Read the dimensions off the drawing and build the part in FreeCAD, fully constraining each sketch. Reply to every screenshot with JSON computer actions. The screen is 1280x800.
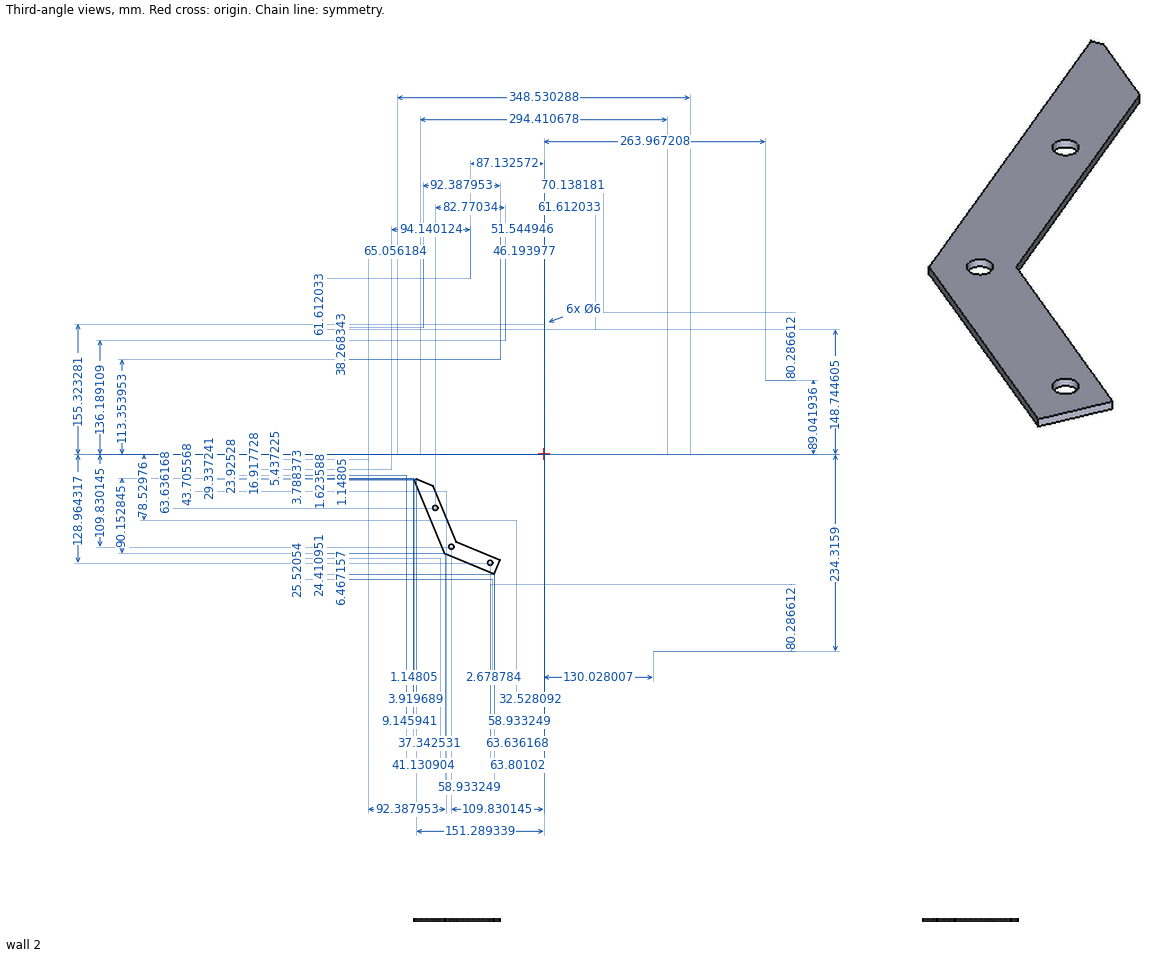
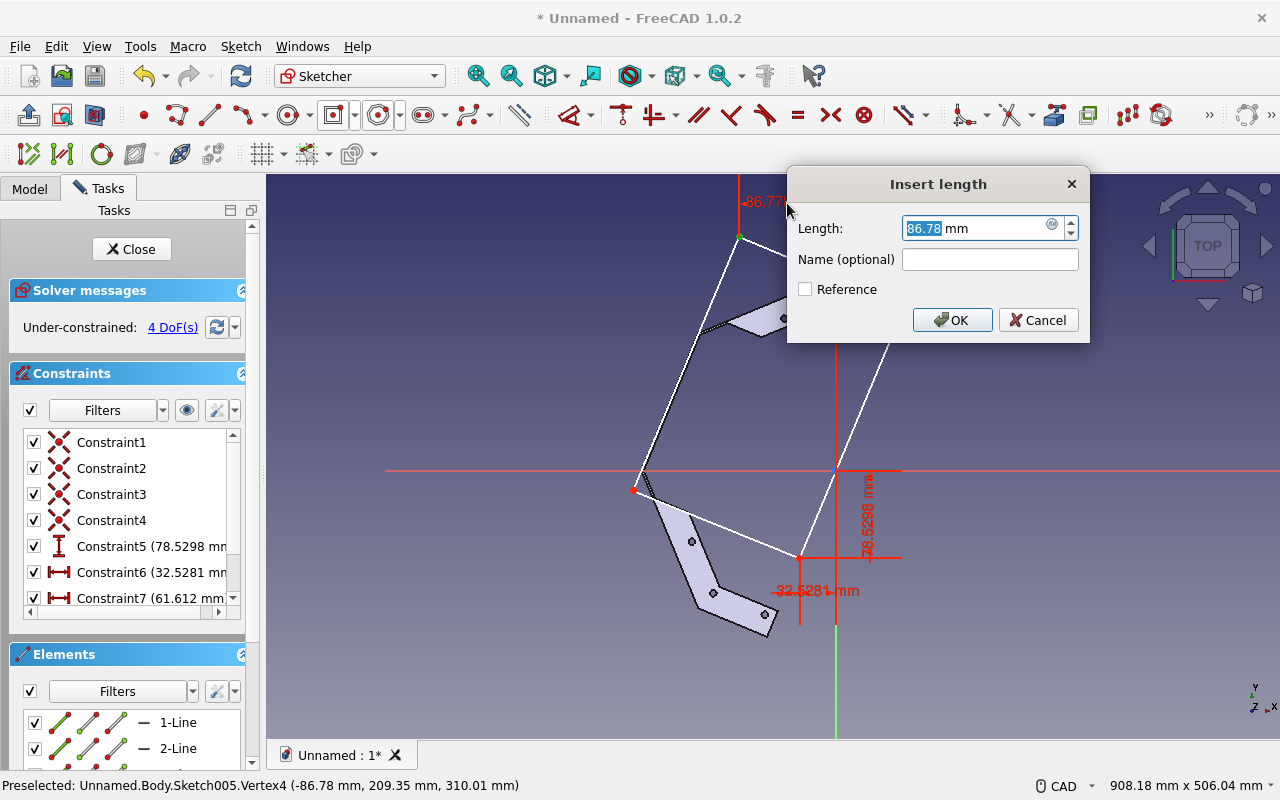
{"action": "type", "text": "87.132572"}
{"action": "key", "text": "Return"}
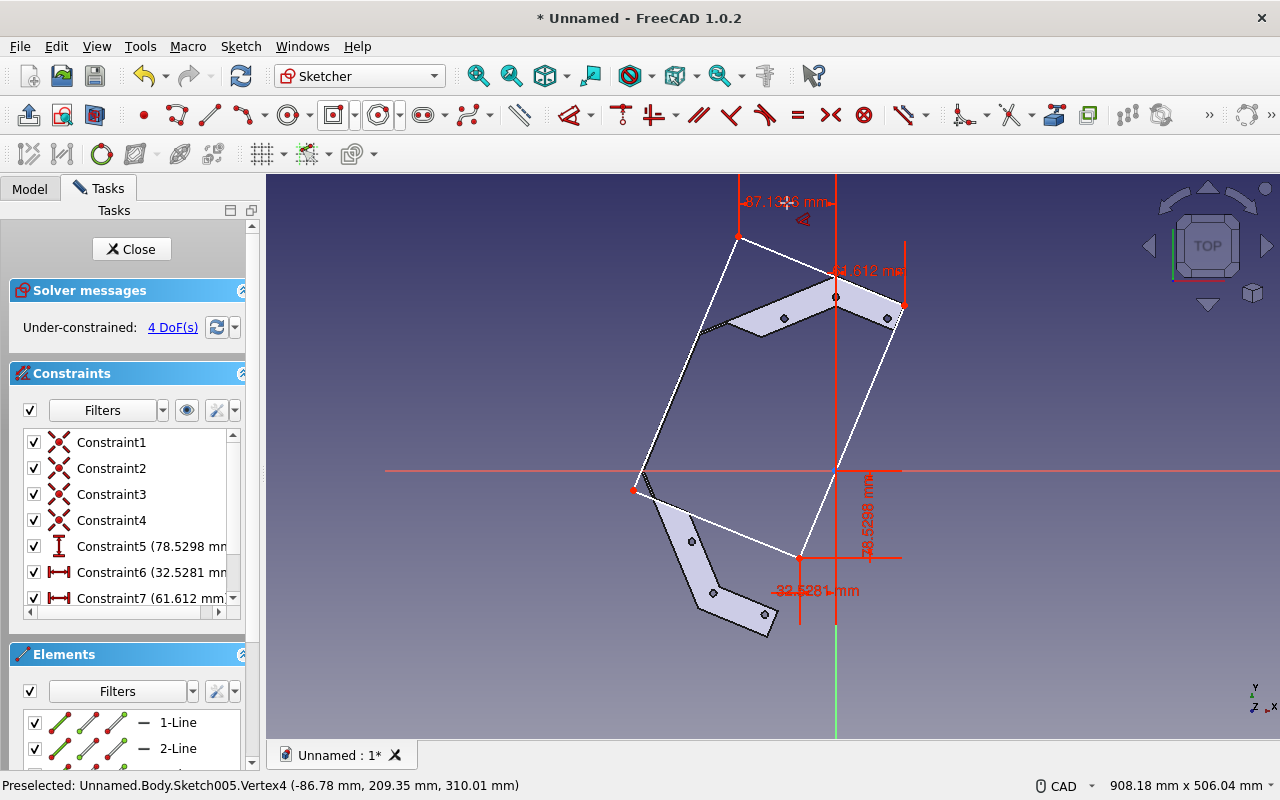
{"action": "scroll", "coordinate": [633, 491], "scroll_direction": "up", "scroll_amount": 4}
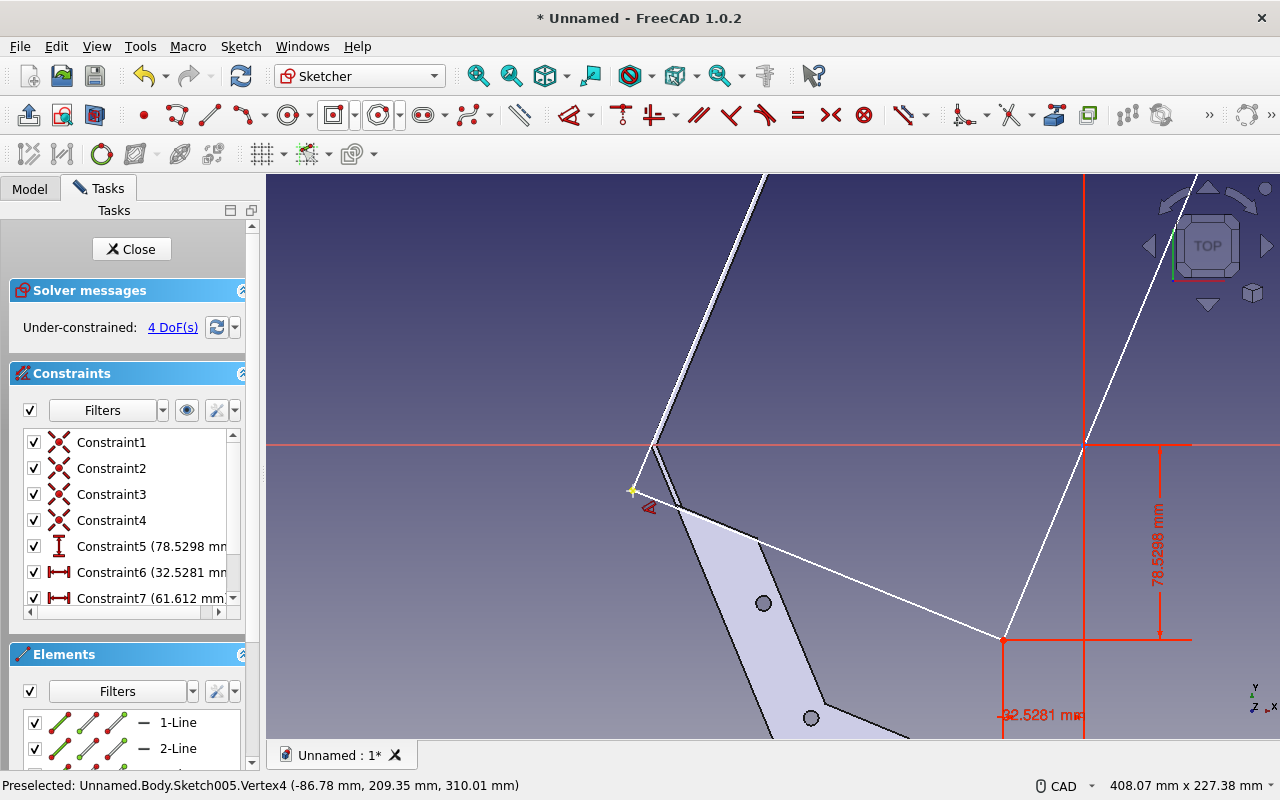
{"action": "left_click", "coordinate": [633, 490]}
{"action": "left_click", "coordinate": [599, 468]}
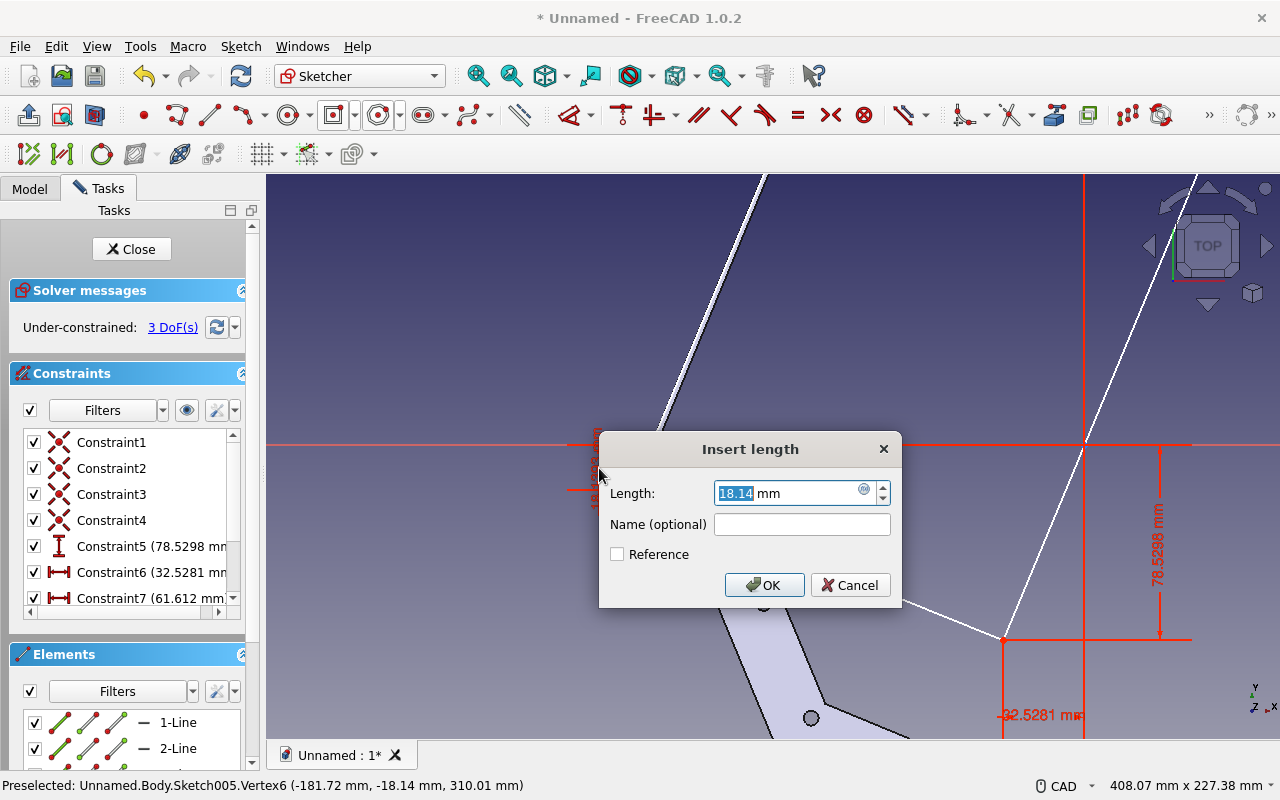
{"action": "type", "text": "16.917728"}
{"action": "key", "text": "Return"}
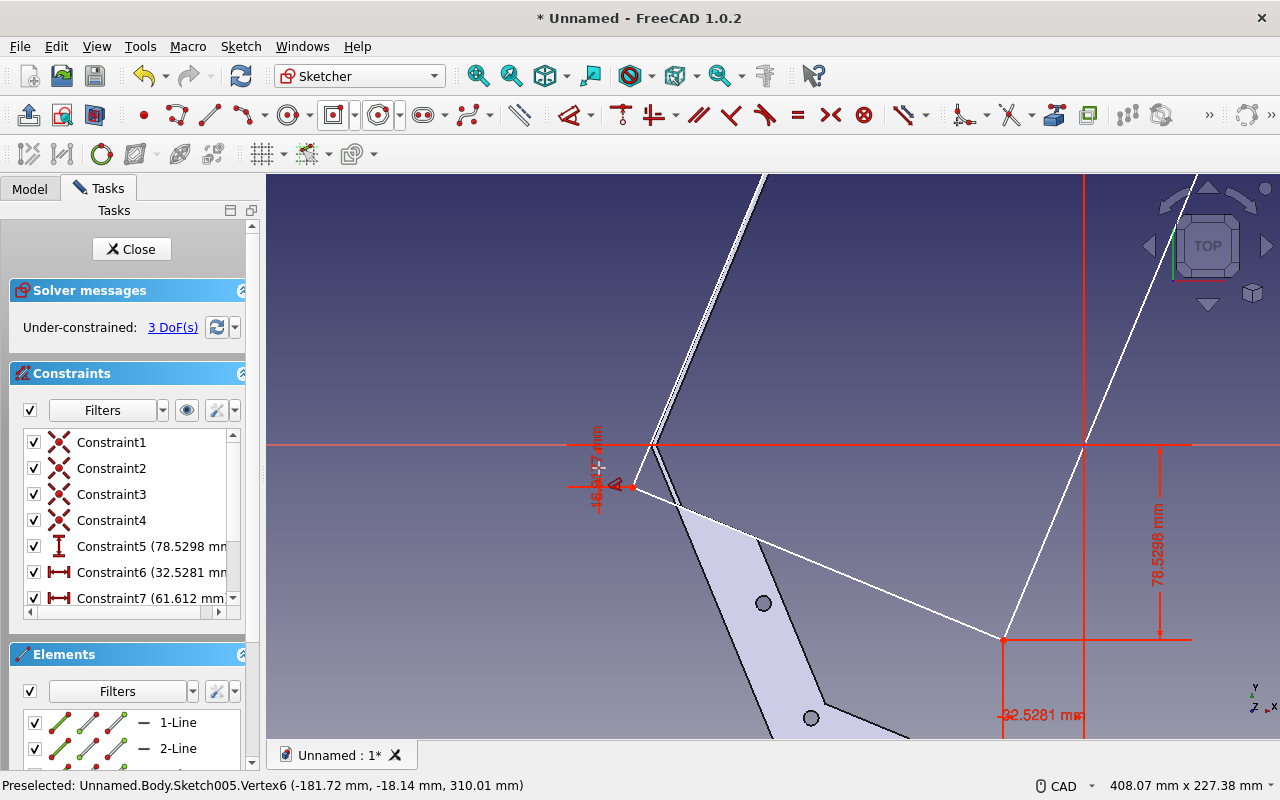
{"action": "scroll", "coordinate": [424, 669], "scroll_direction": "down", "scroll_amount": 3}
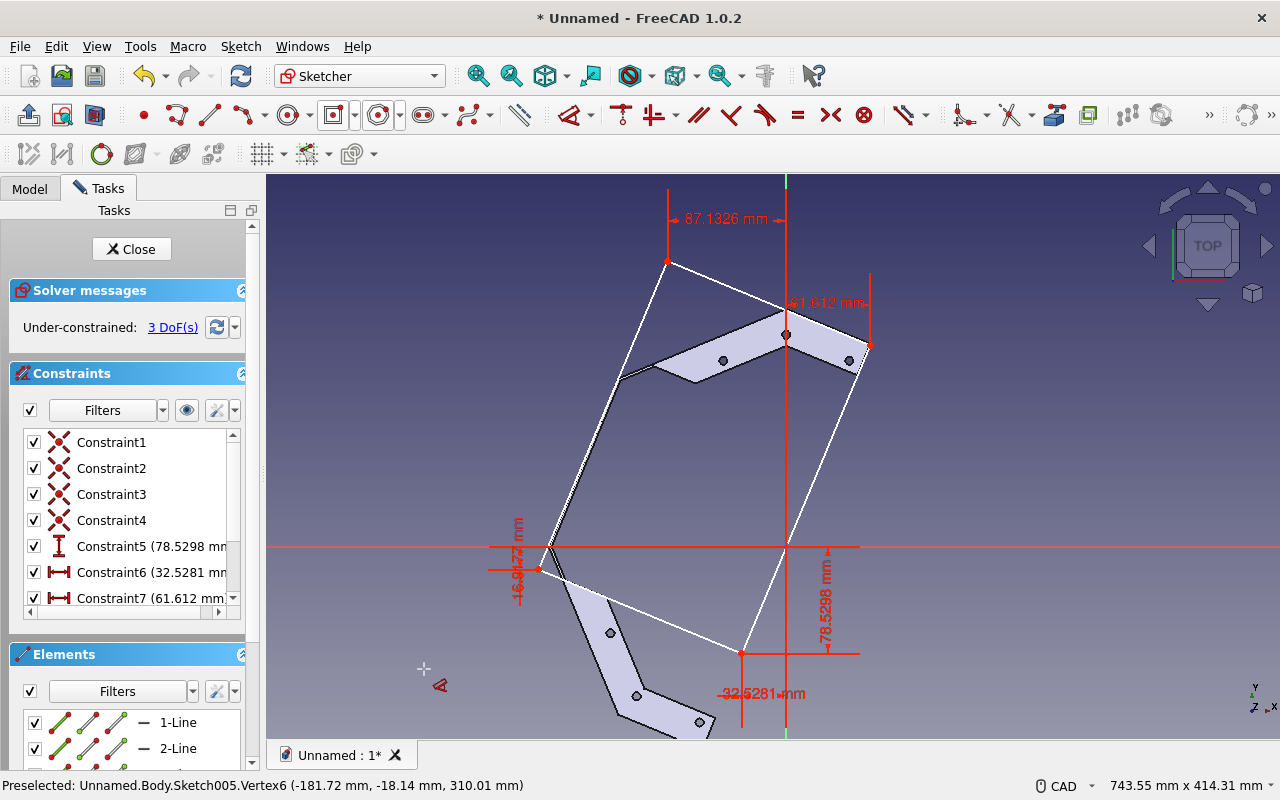
{"action": "left_click", "coordinate": [810, 320]}
{"action": "left_click", "coordinate": [904, 303]}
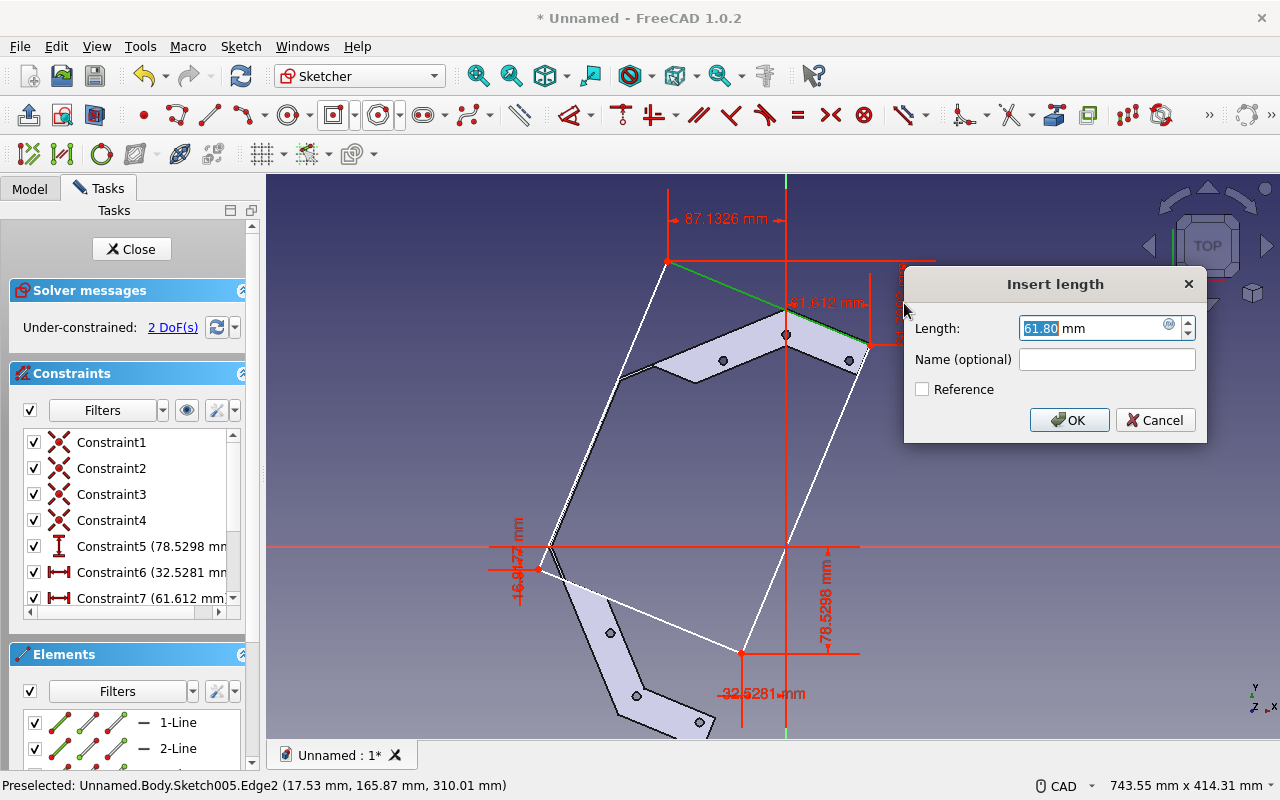
{"action": "type", "text": "61.612033"}
{"action": "key", "text": "Return"}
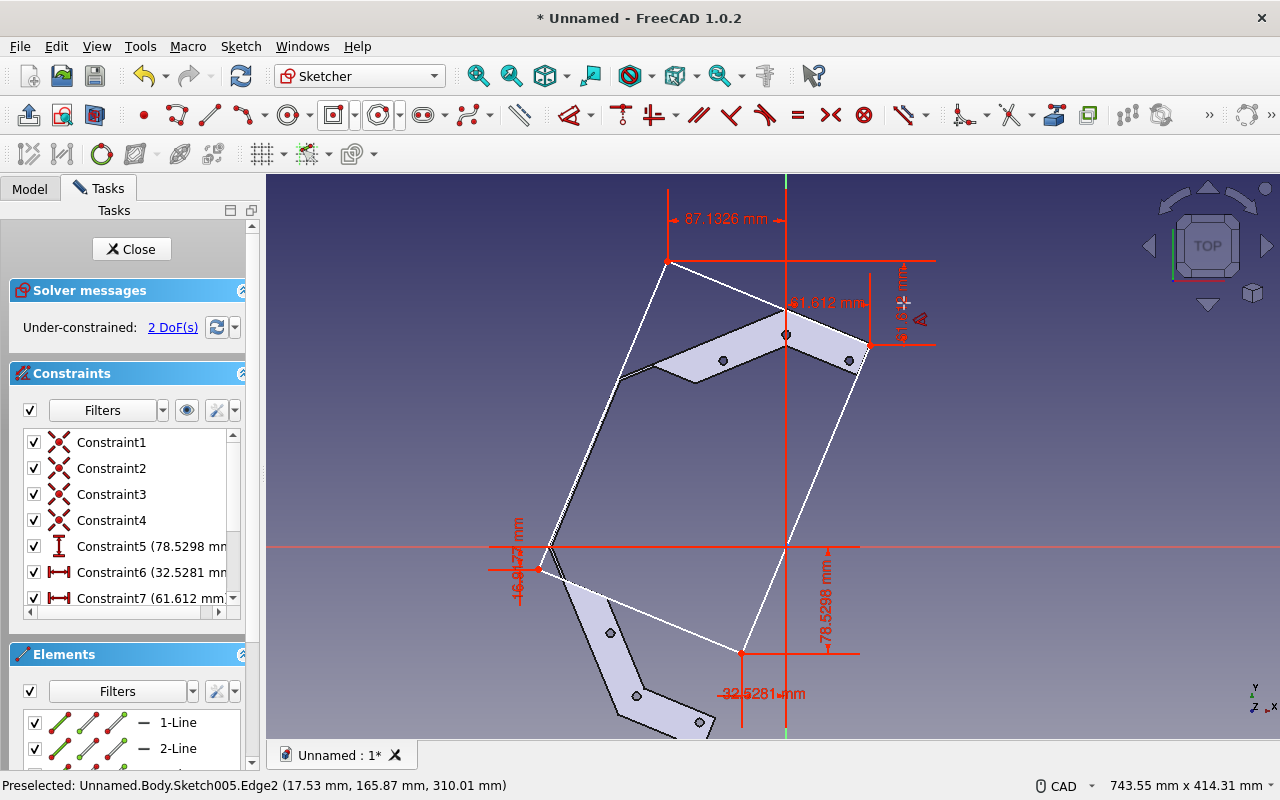
{"action": "left_click", "coordinate": [629, 354]}
{"action": "left_click", "coordinate": [603, 227]}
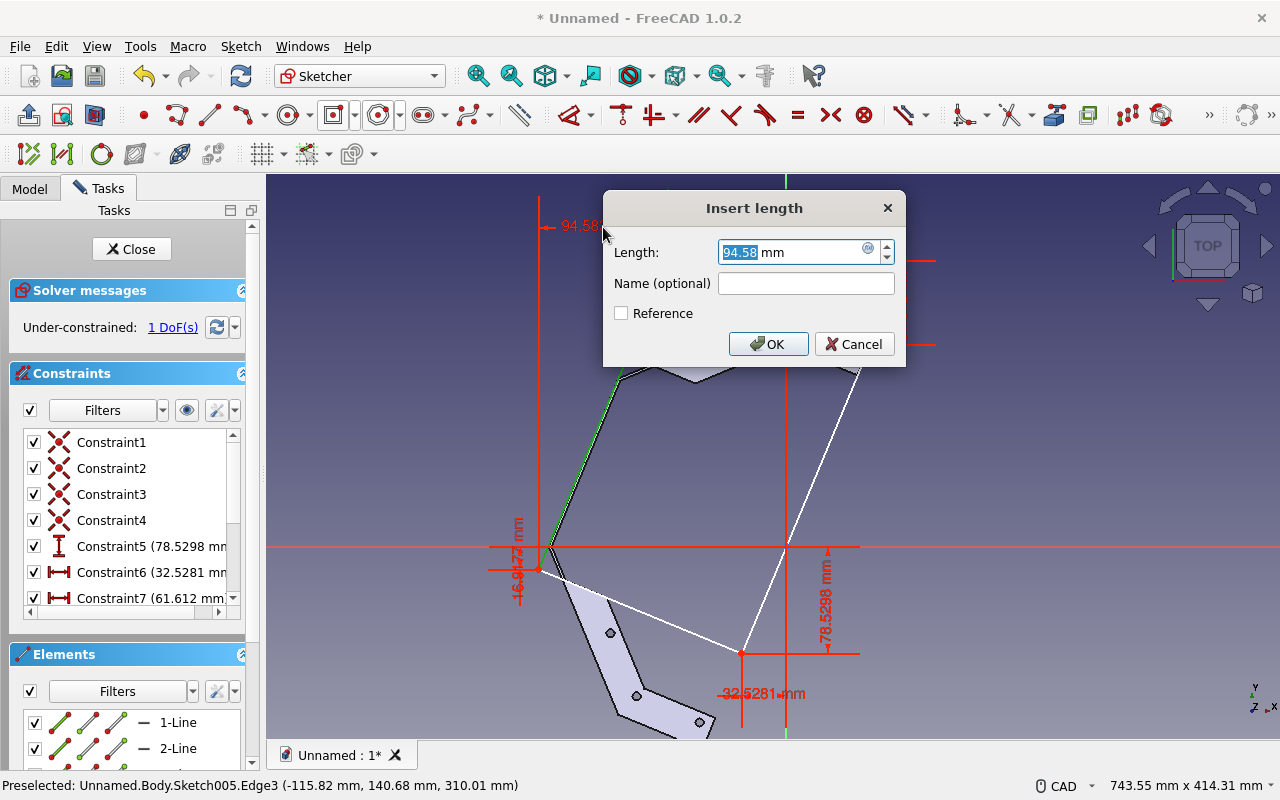
{"action": "type", "text": "94.140124"}
{"action": "key", "text": "Return"}